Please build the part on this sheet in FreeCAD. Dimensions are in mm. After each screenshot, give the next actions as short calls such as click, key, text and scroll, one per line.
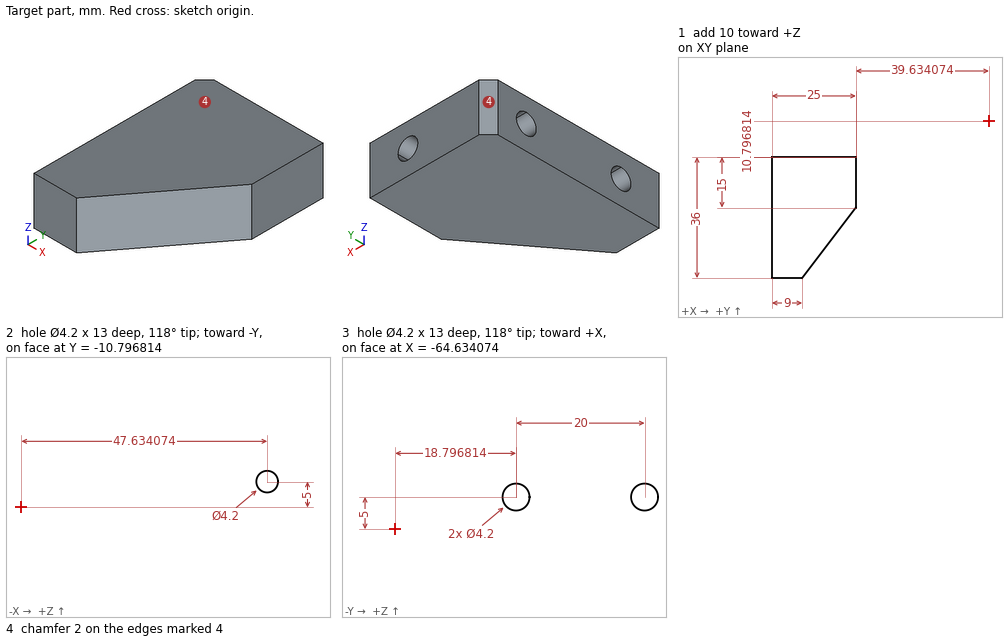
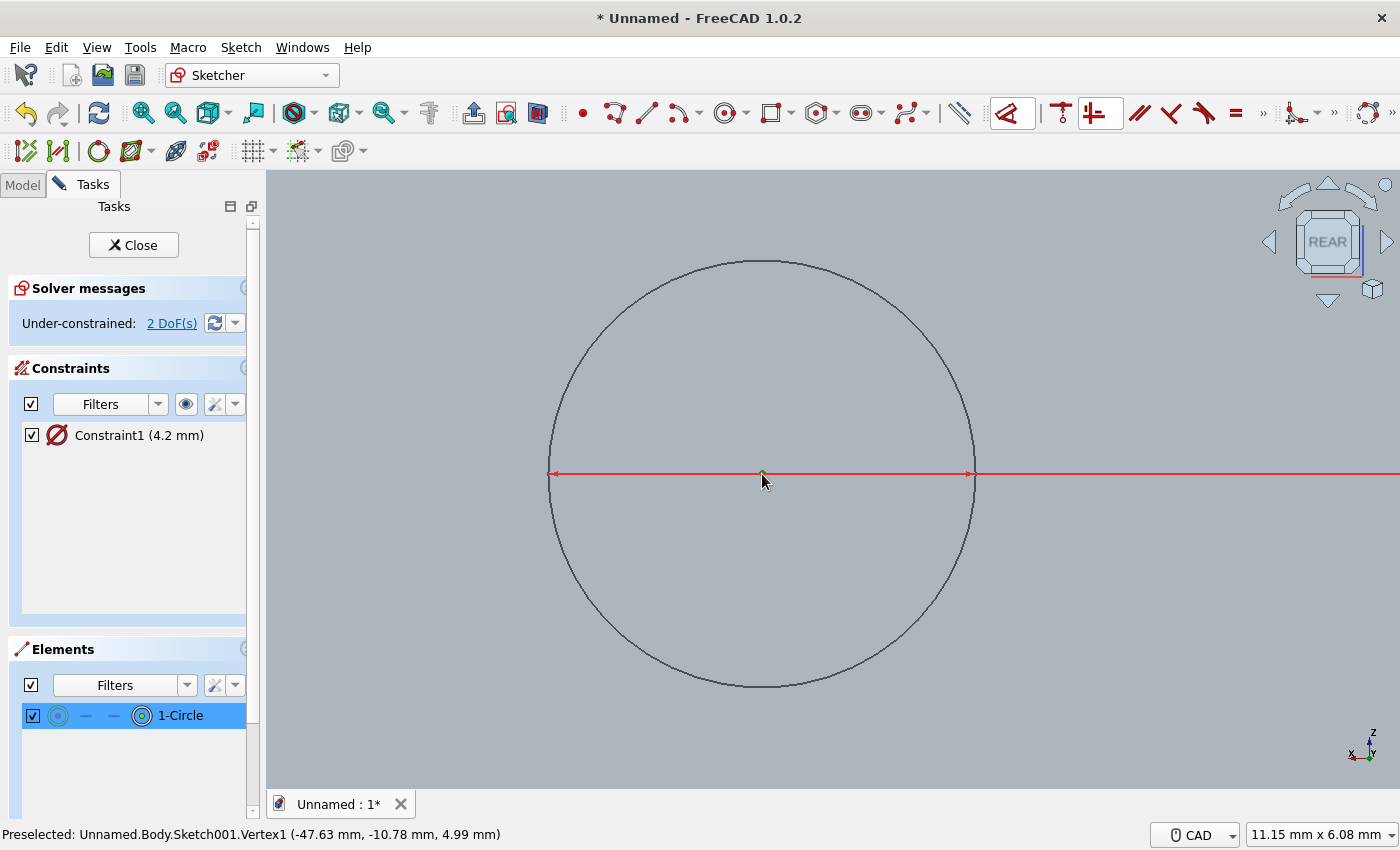
key(i)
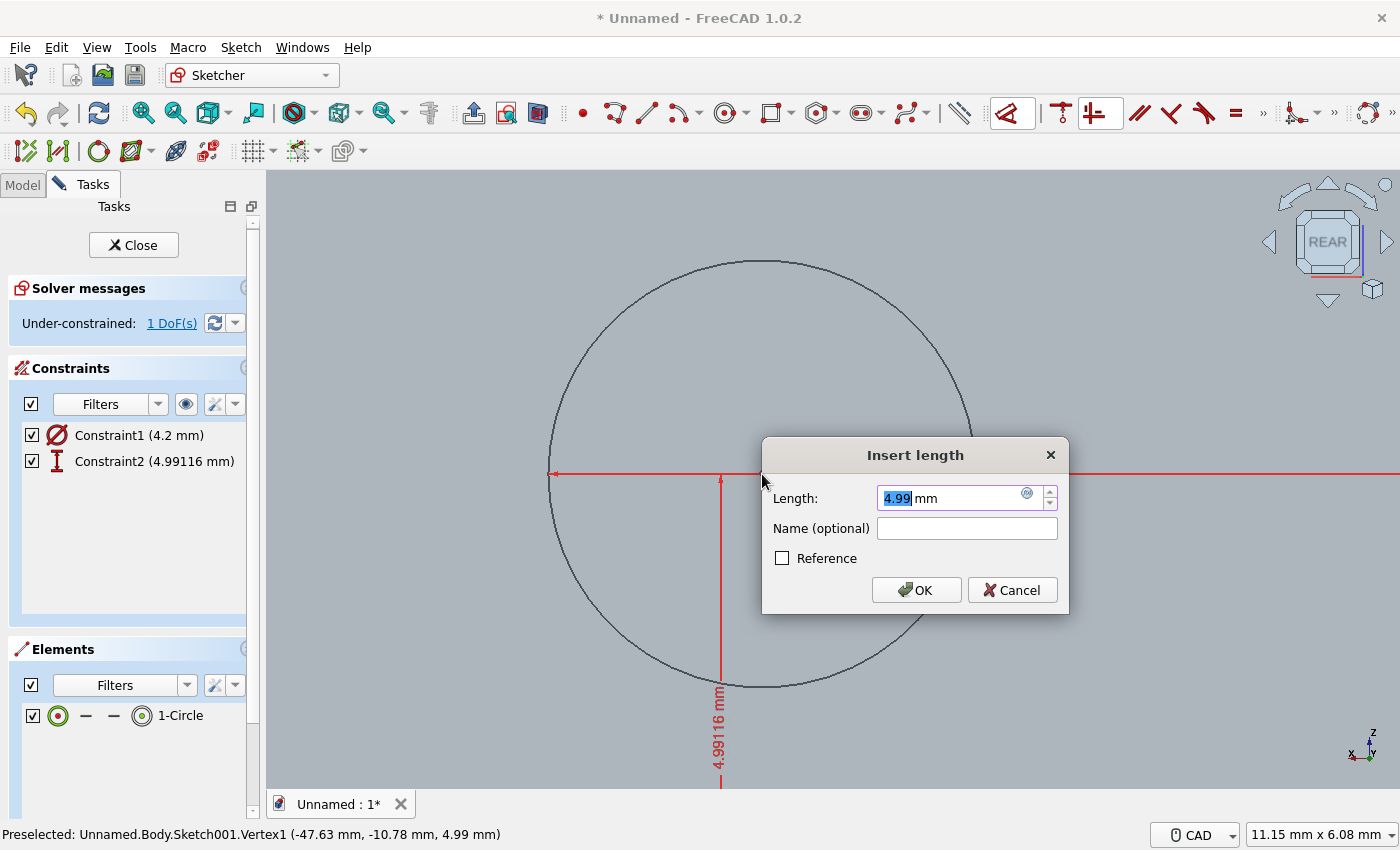
text(5)
key(Return)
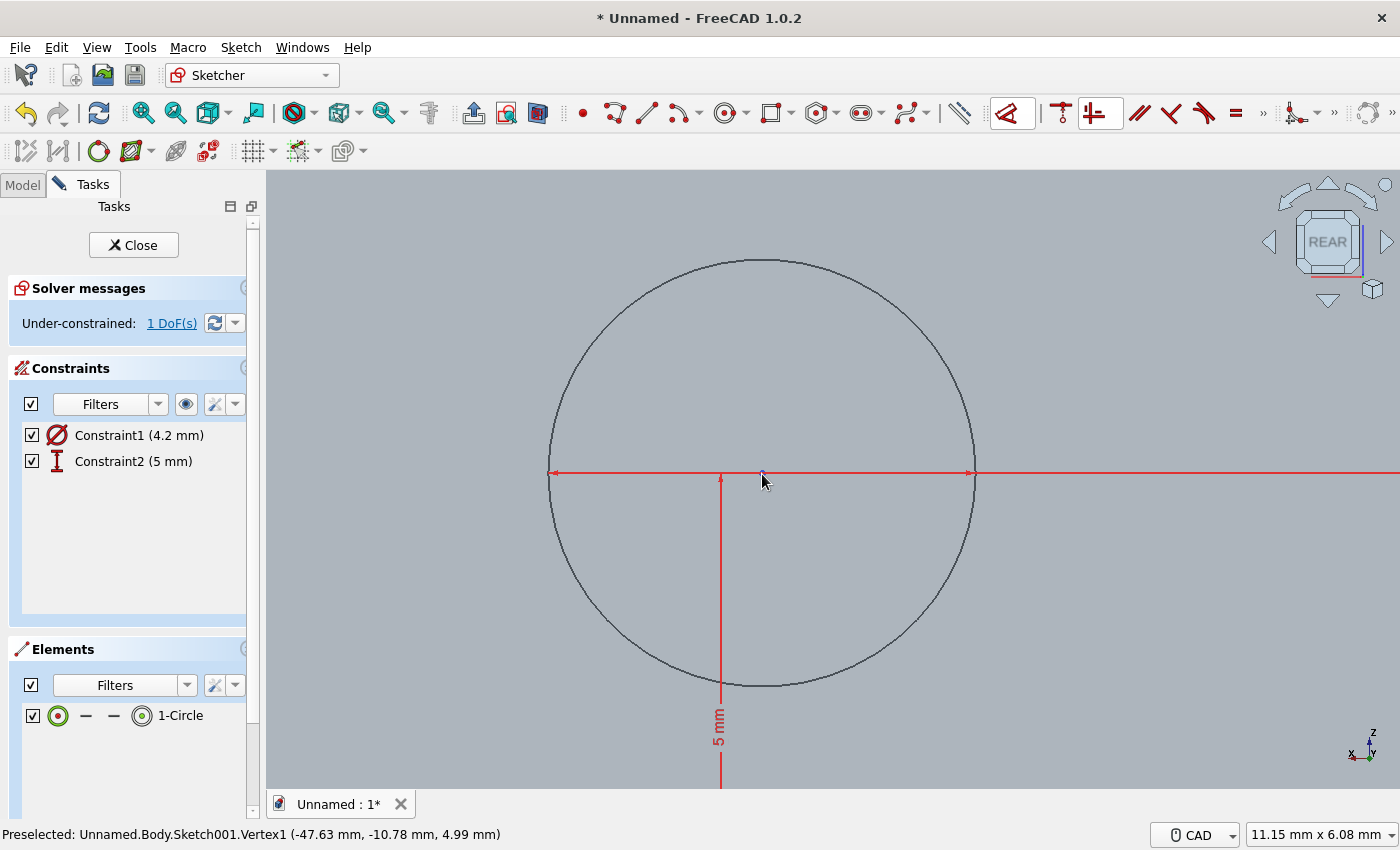
click(762, 473)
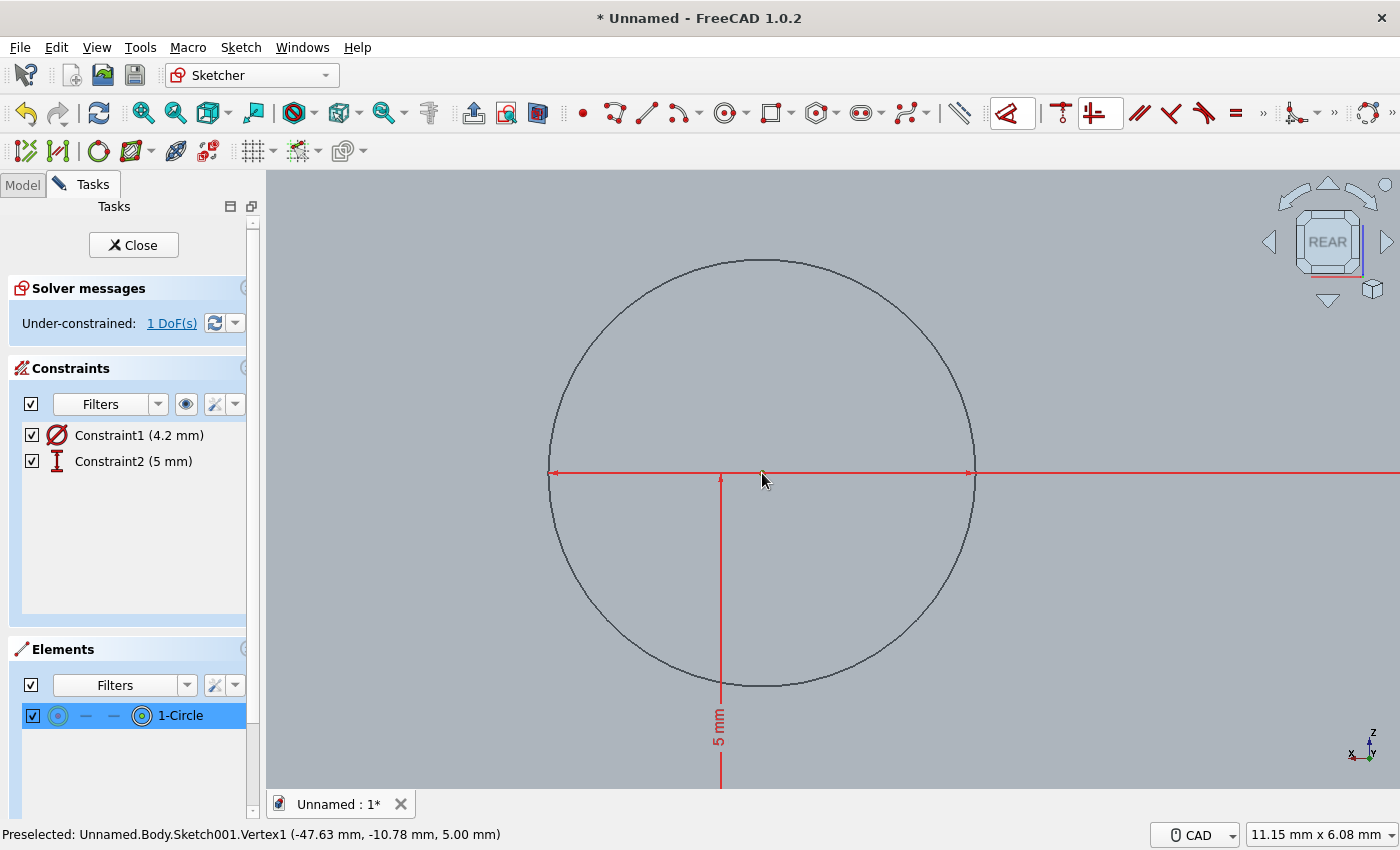
click(1030, 114)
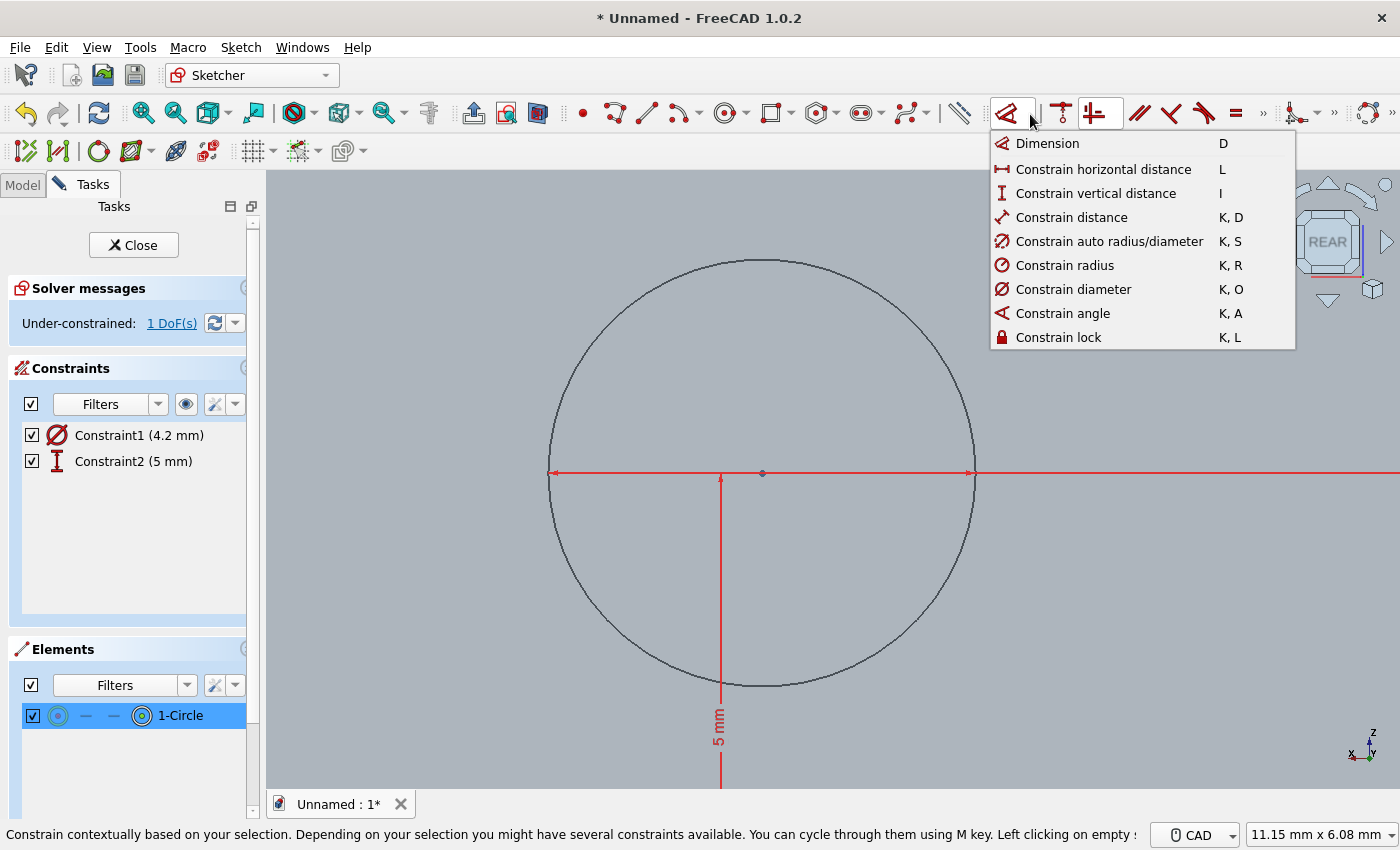
click(1143, 169)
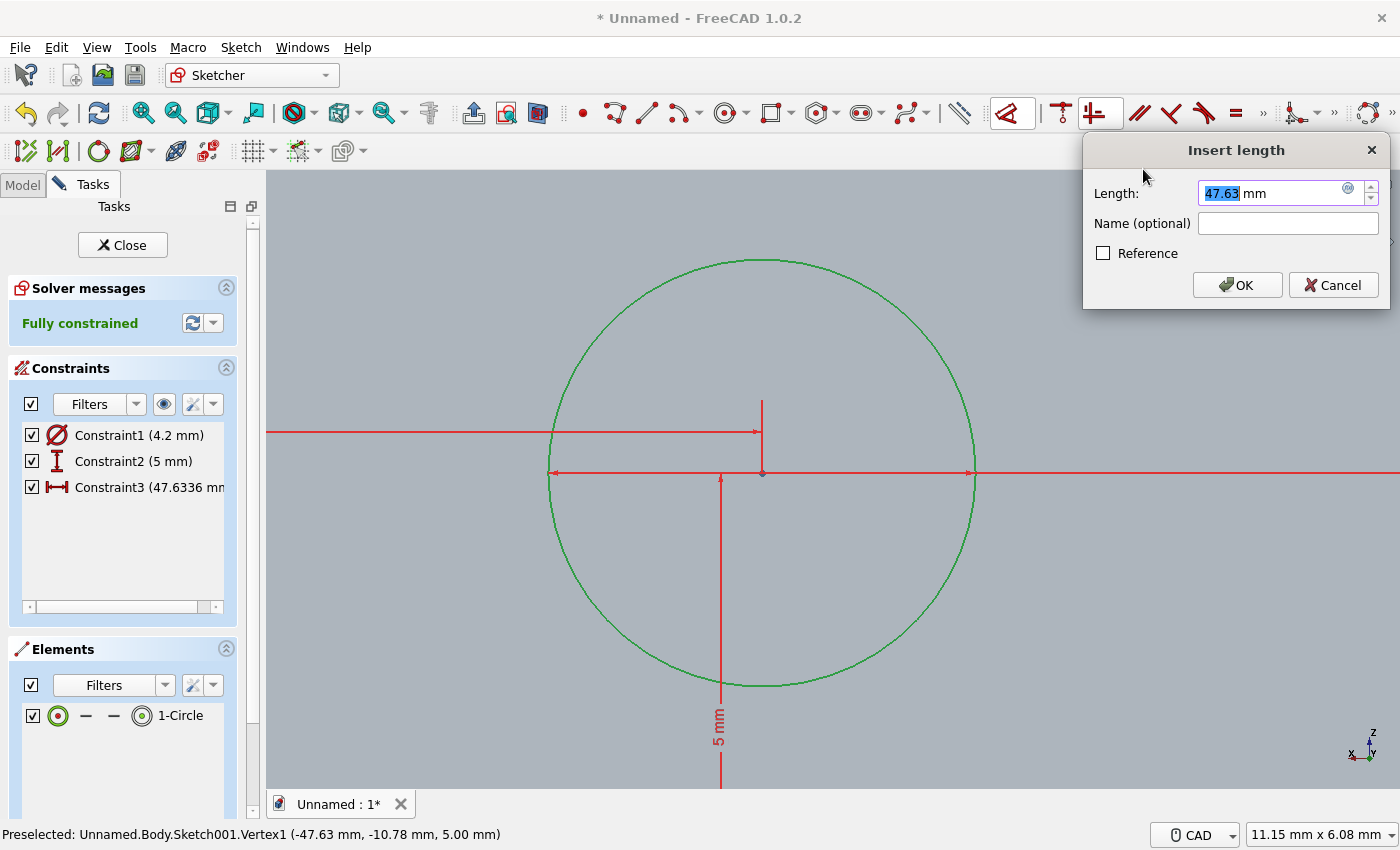
text(47.634074)
key(Return)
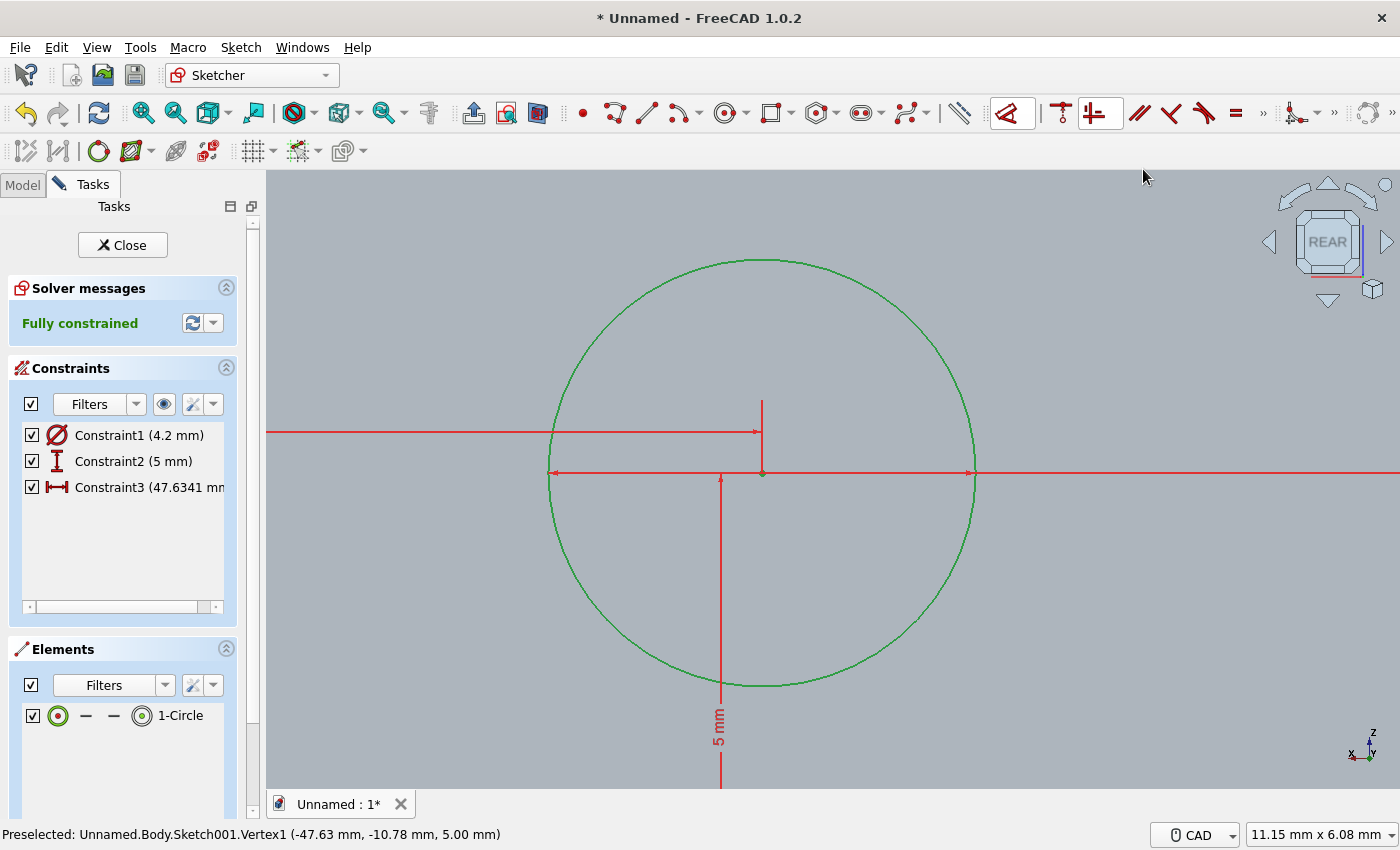
click(123, 245)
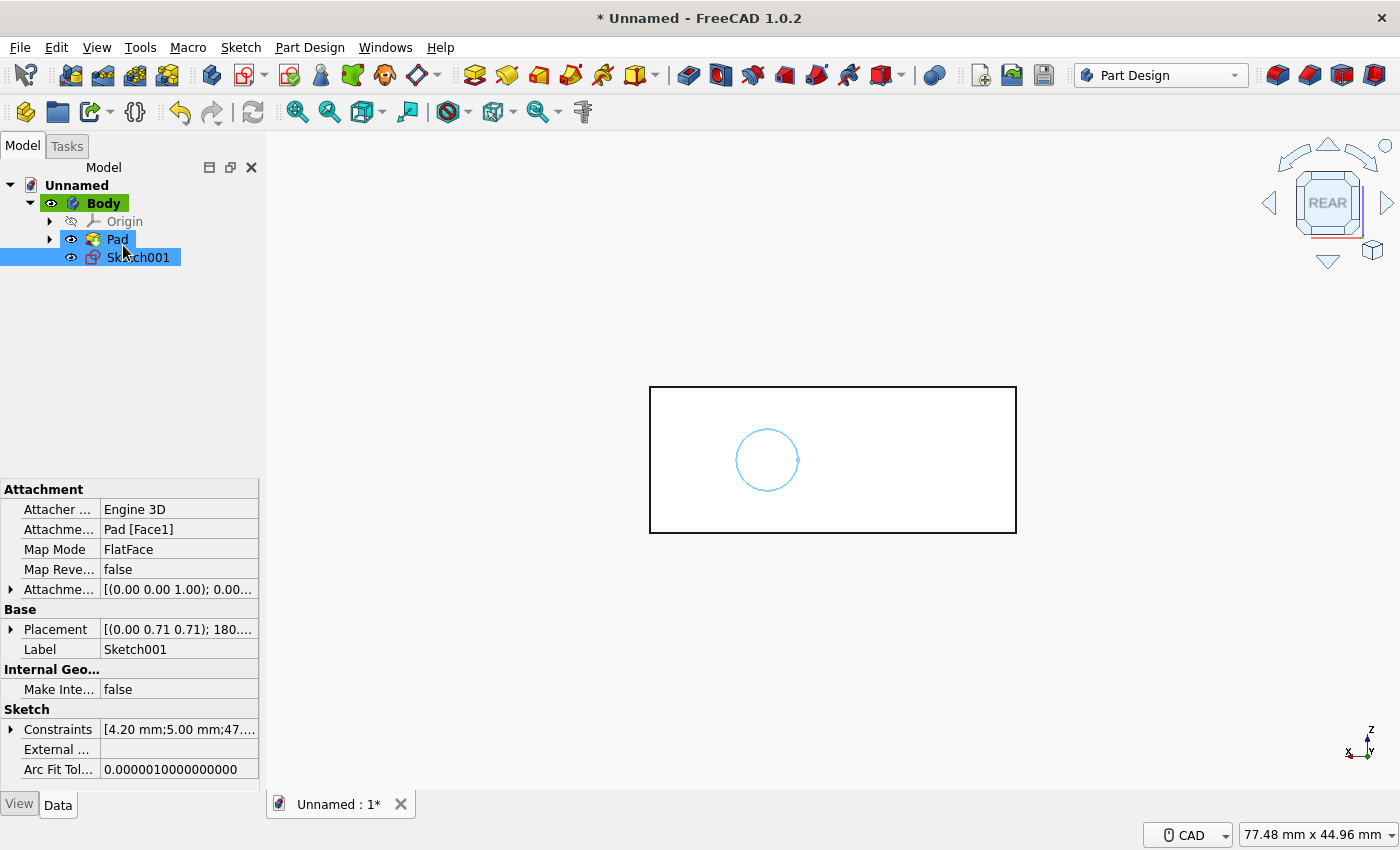
click(722, 76)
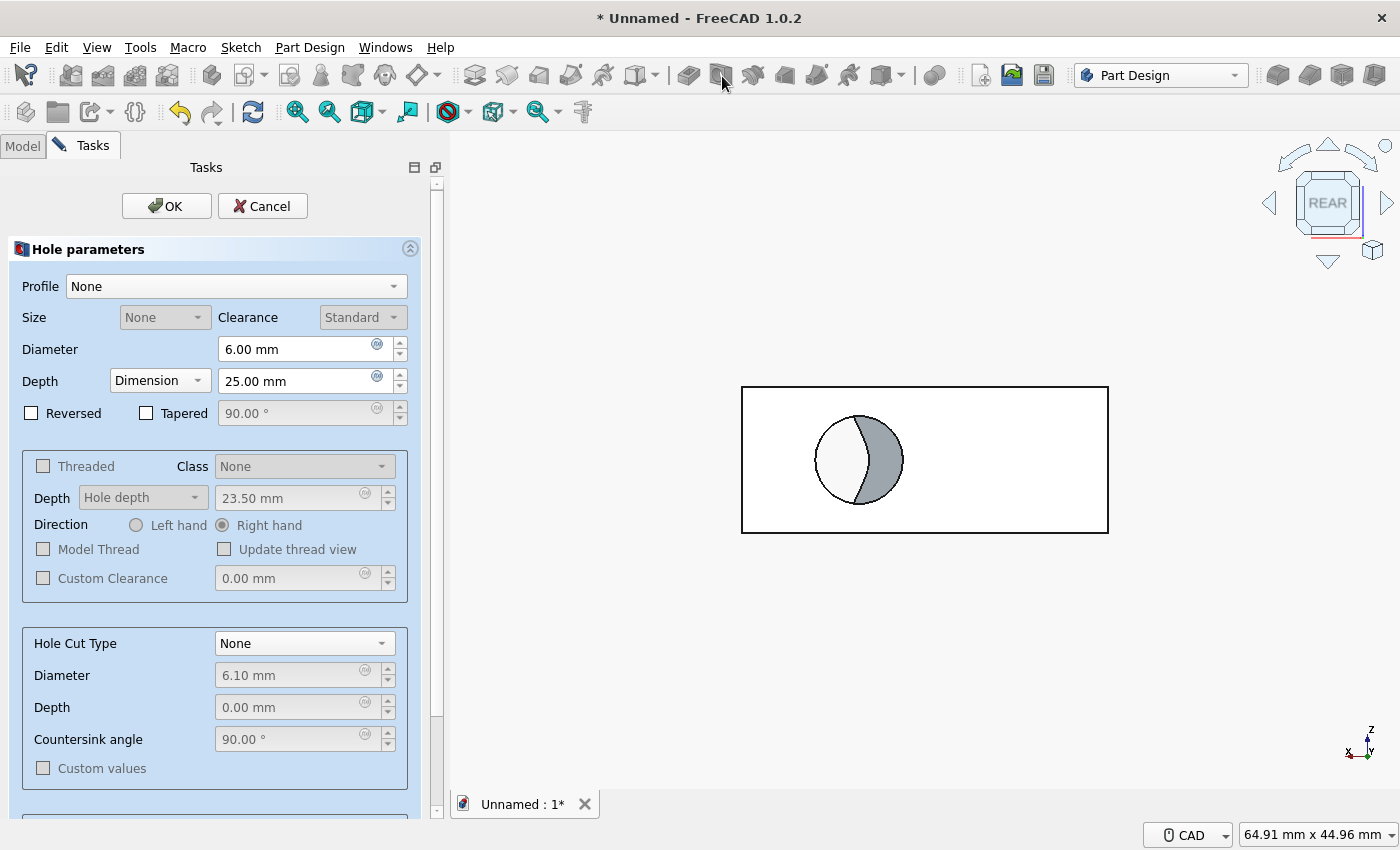
triple_click(305, 349)